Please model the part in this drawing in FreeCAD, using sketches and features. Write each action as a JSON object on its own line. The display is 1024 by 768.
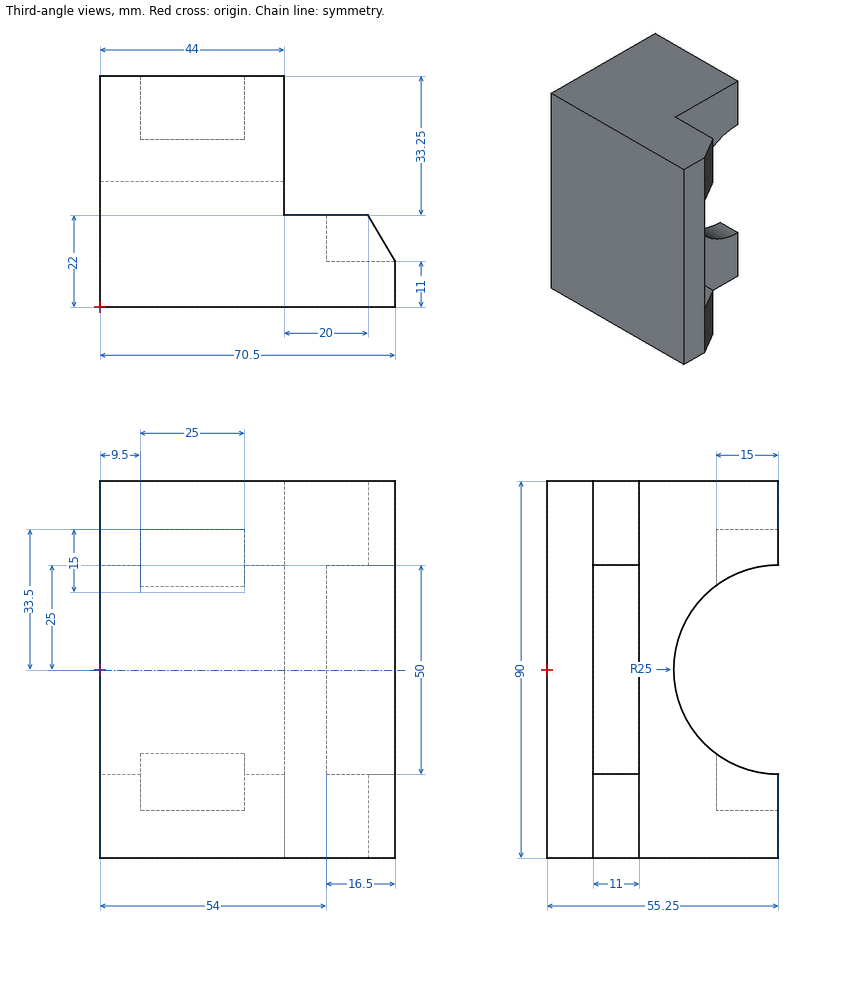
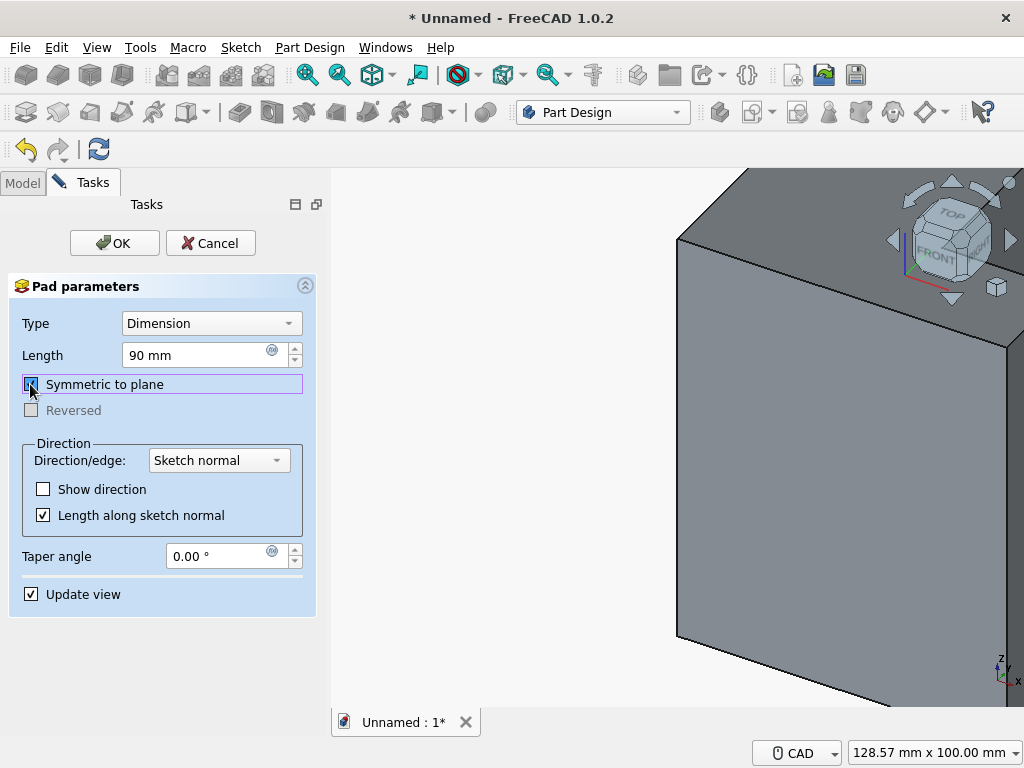
{"action": "left_click", "coordinate": [115, 243]}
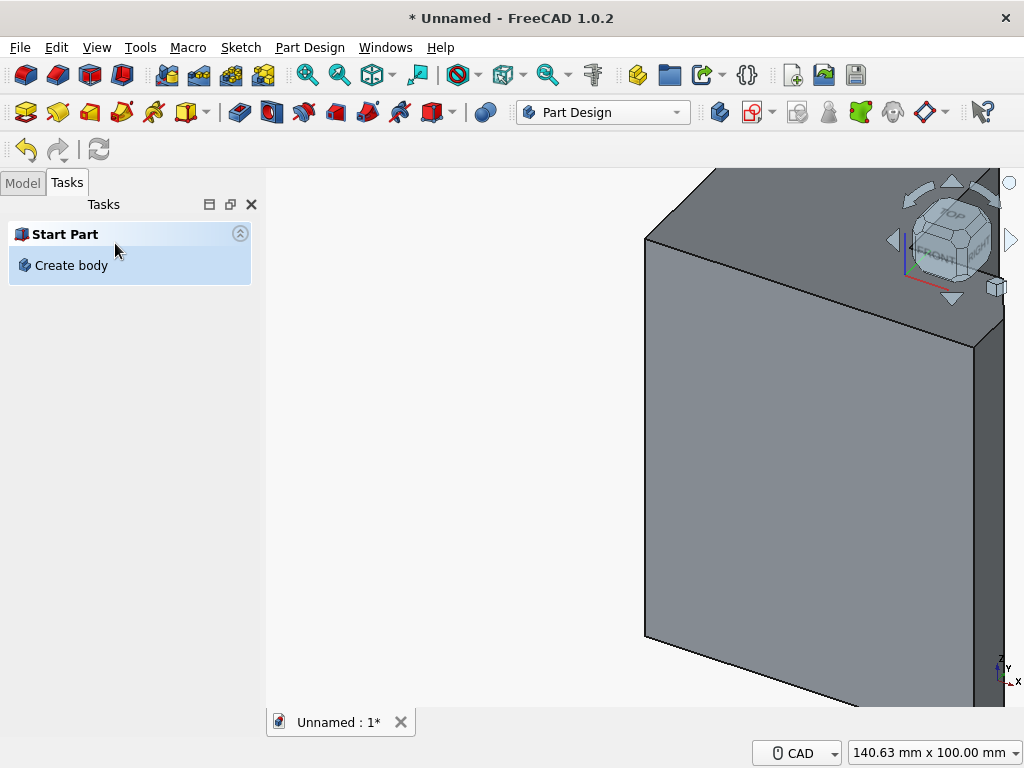
{"action": "key", "text": "v f"}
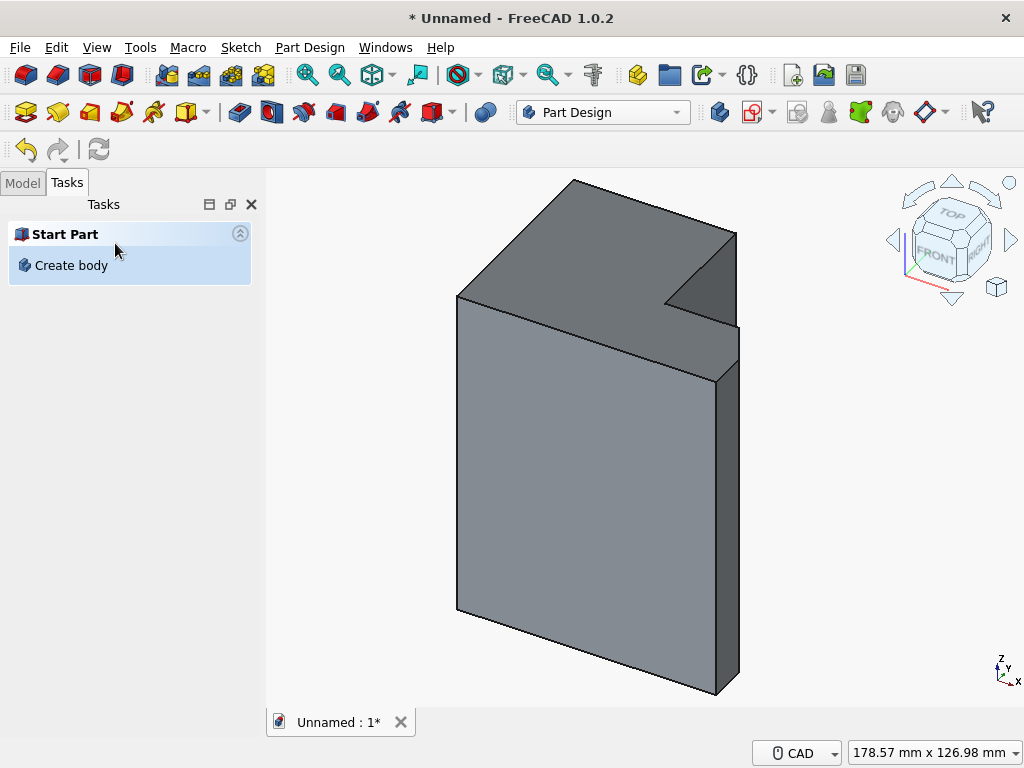
{"action": "key", "text": "0"}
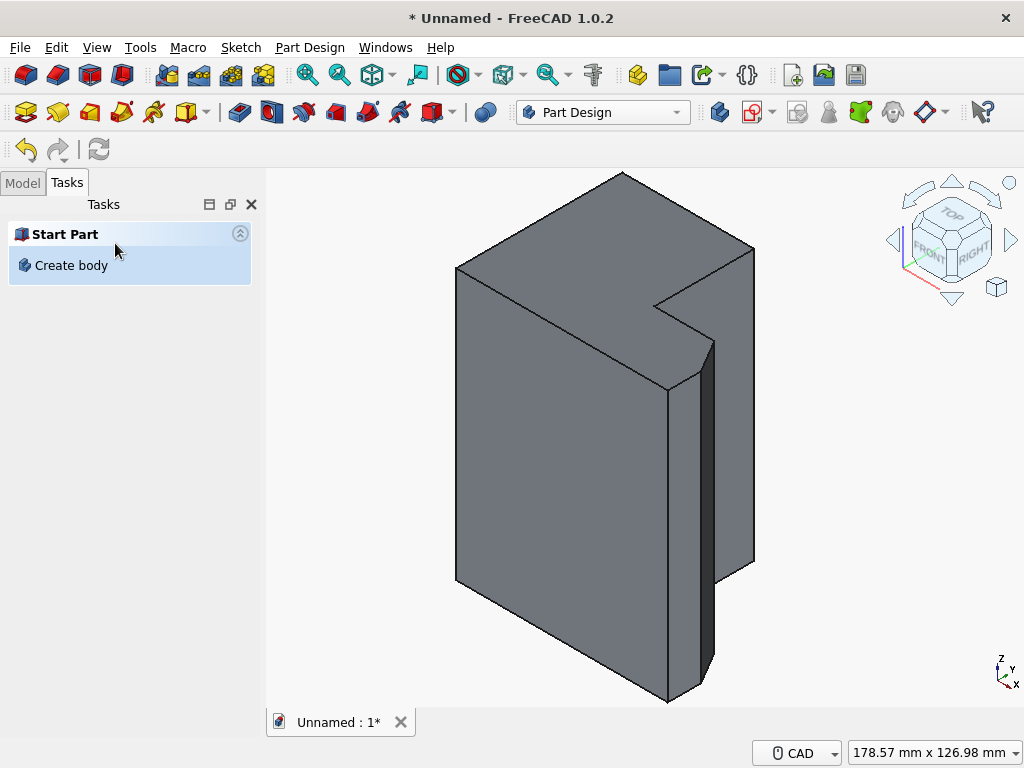
{"action": "key", "text": "3"}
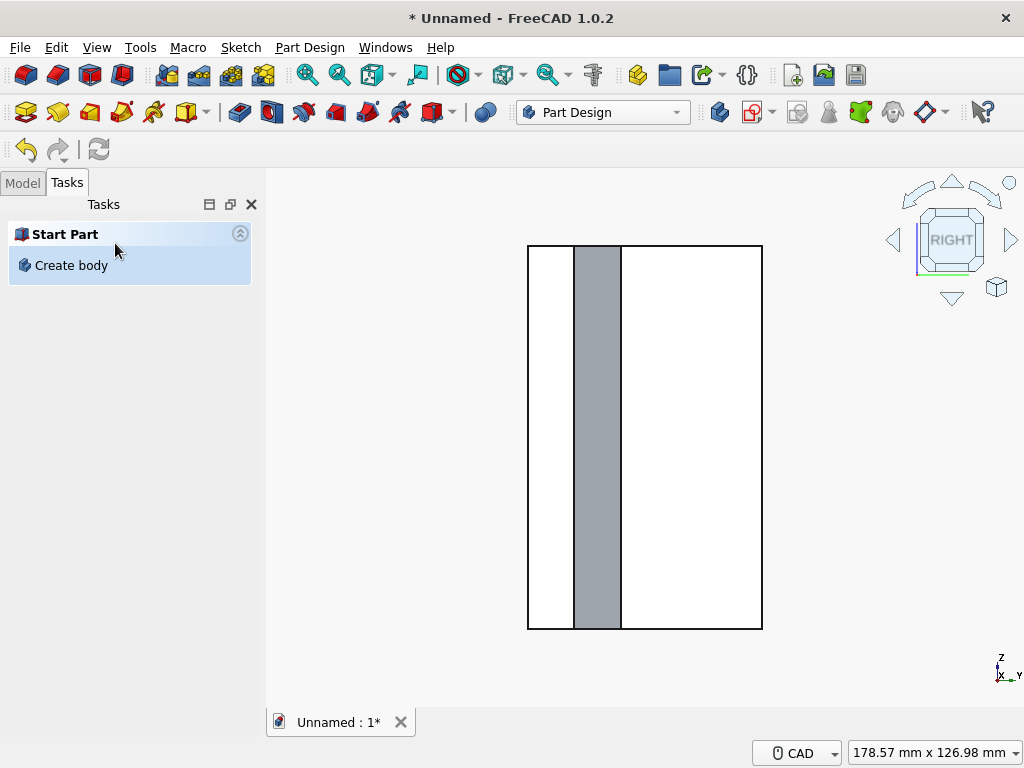
{"action": "left_click", "coordinate": [692, 327]}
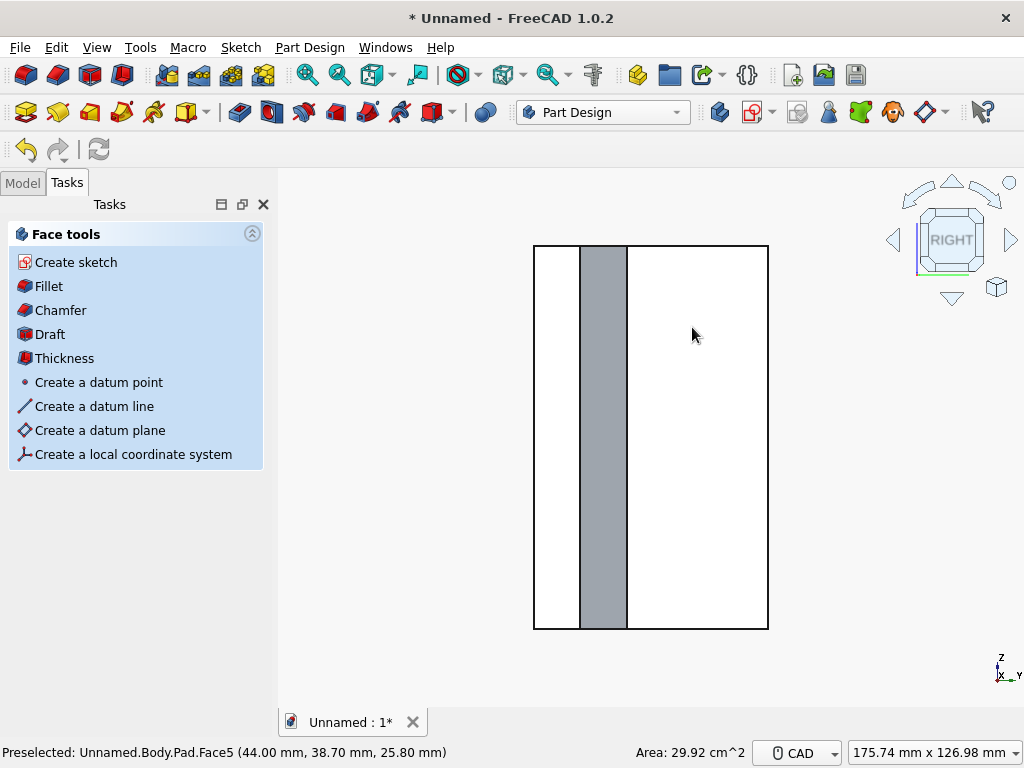
{"action": "left_click", "coordinate": [752, 112]}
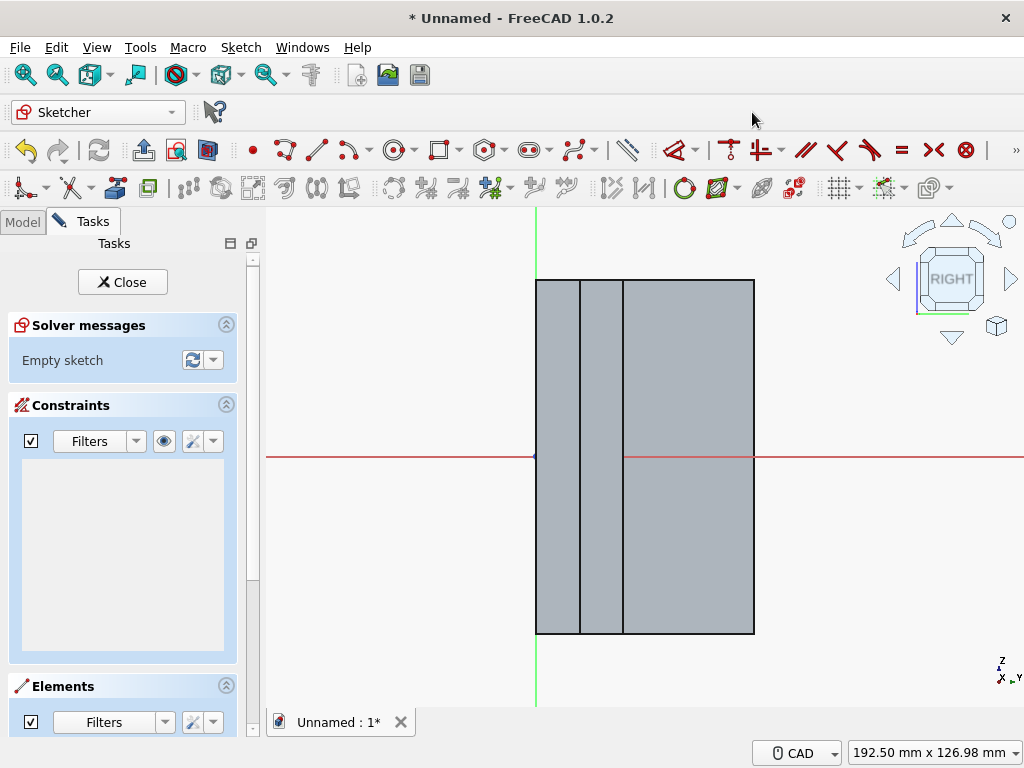
{"action": "scroll", "coordinate": [784, 457], "scroll_direction": "up", "scroll_amount": 2}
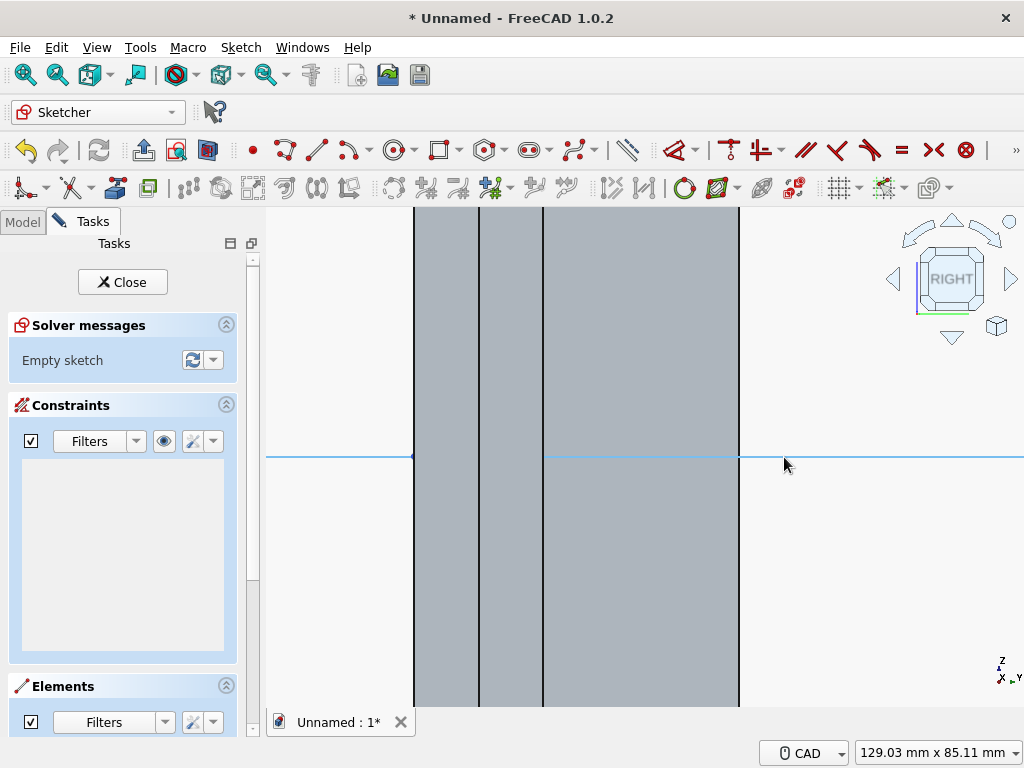
{"action": "key", "text": "g l"}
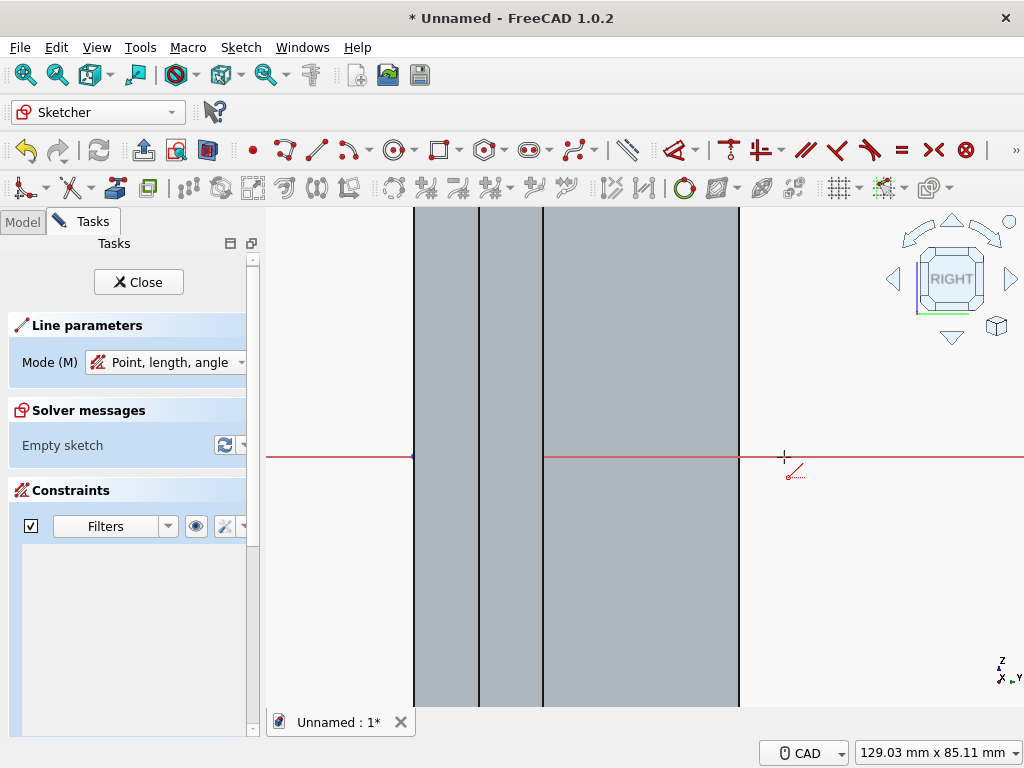
{"action": "left_click", "coordinate": [739, 604]}
{"action": "left_click", "coordinate": [739, 310]}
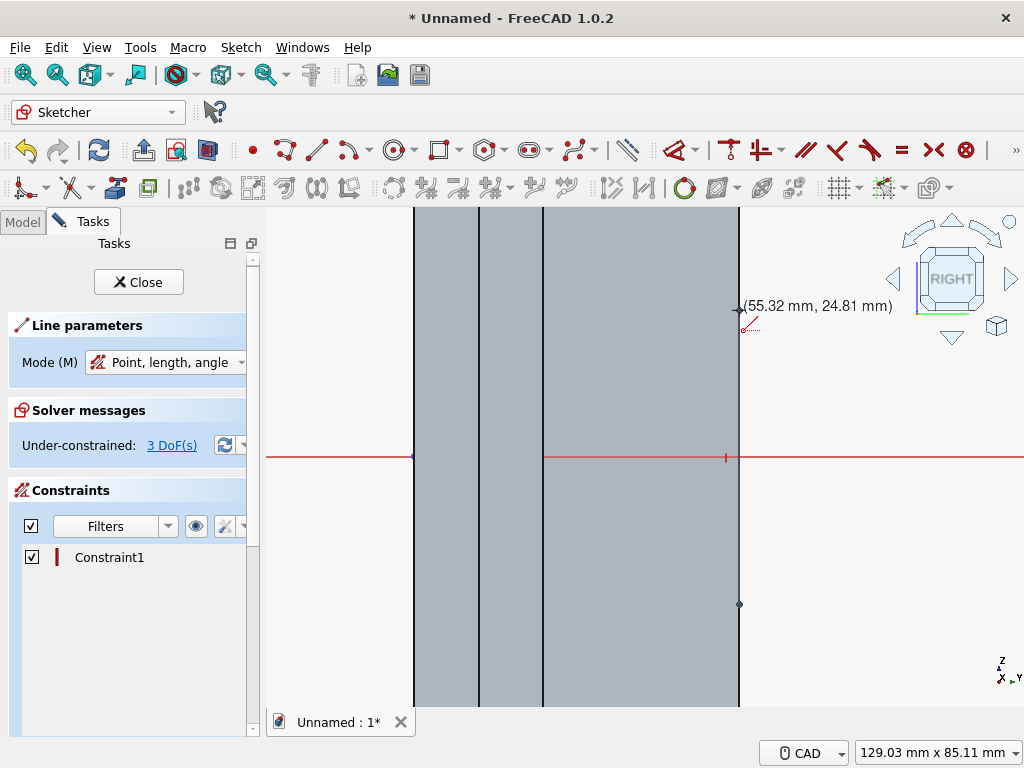
{"action": "left_click", "coordinate": [372, 150]}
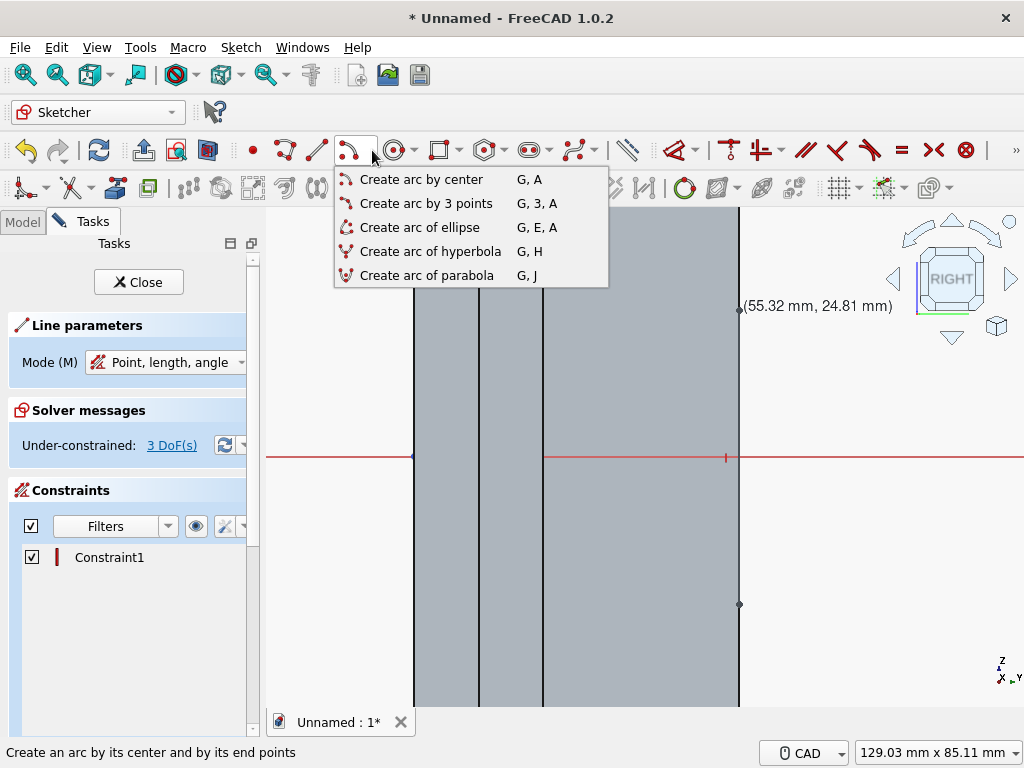
{"action": "left_click", "coordinate": [472, 203]}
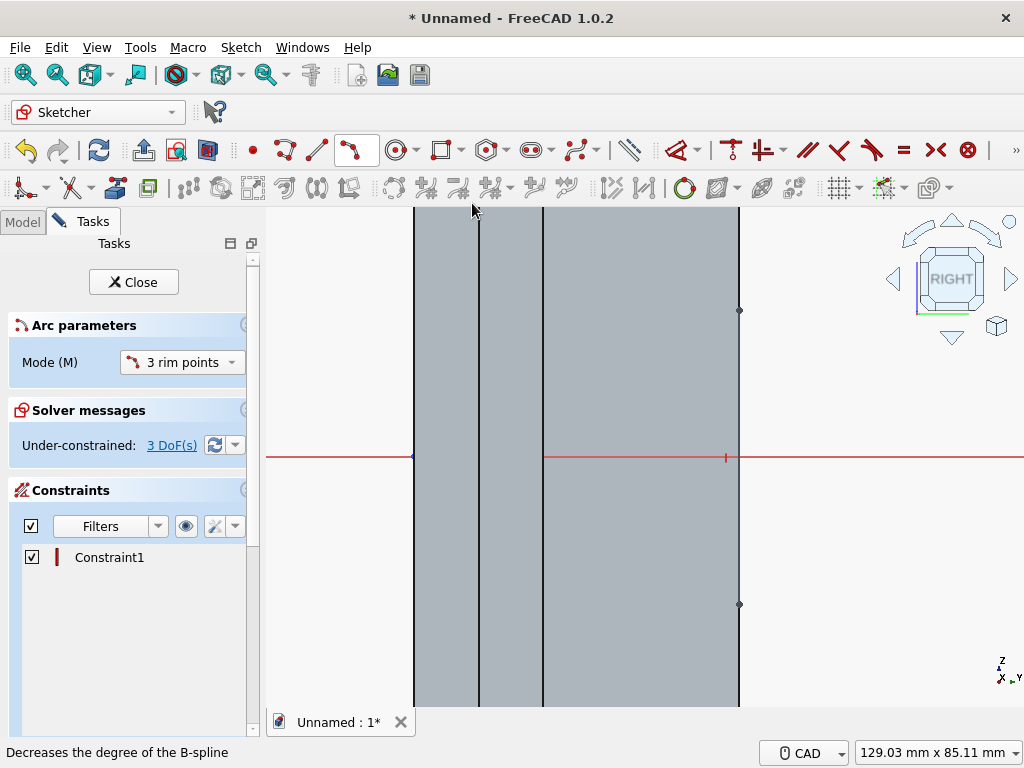
{"action": "left_click", "coordinate": [739, 311]}
{"action": "left_click", "coordinate": [739, 605]}
{"action": "left_click", "coordinate": [599, 411]}
{"action": "key", "text": "Escape"}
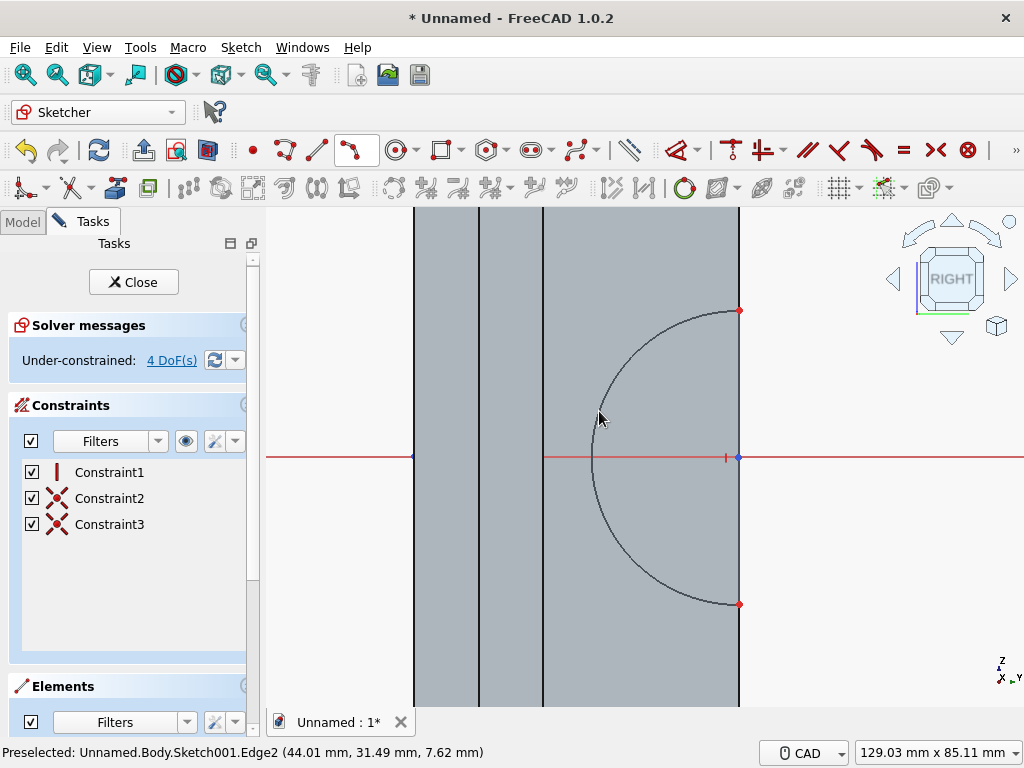
{"action": "left_click", "coordinate": [739, 458]}